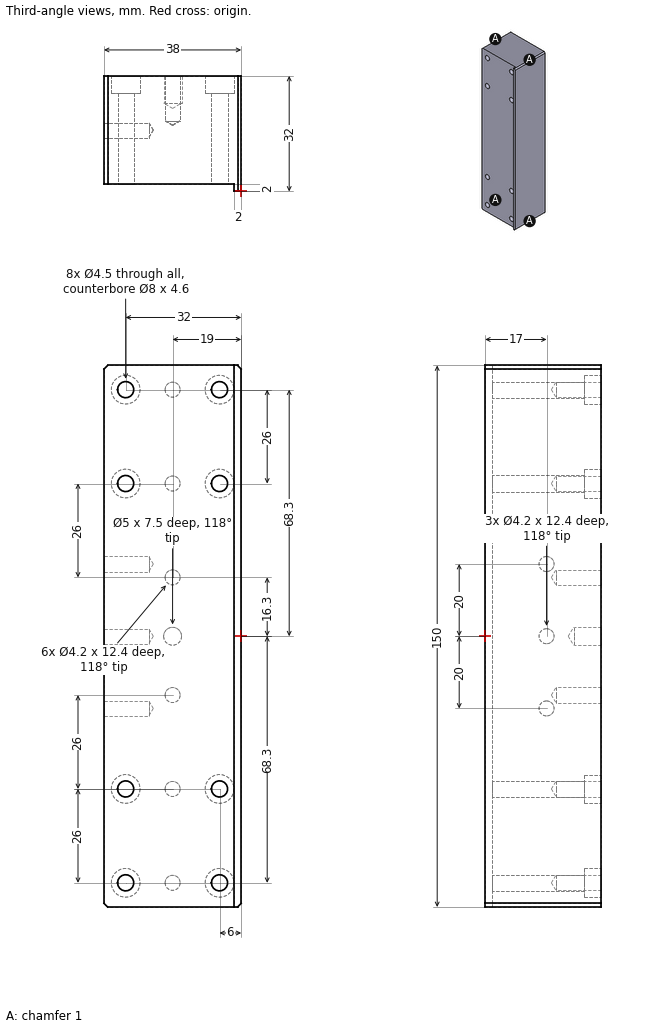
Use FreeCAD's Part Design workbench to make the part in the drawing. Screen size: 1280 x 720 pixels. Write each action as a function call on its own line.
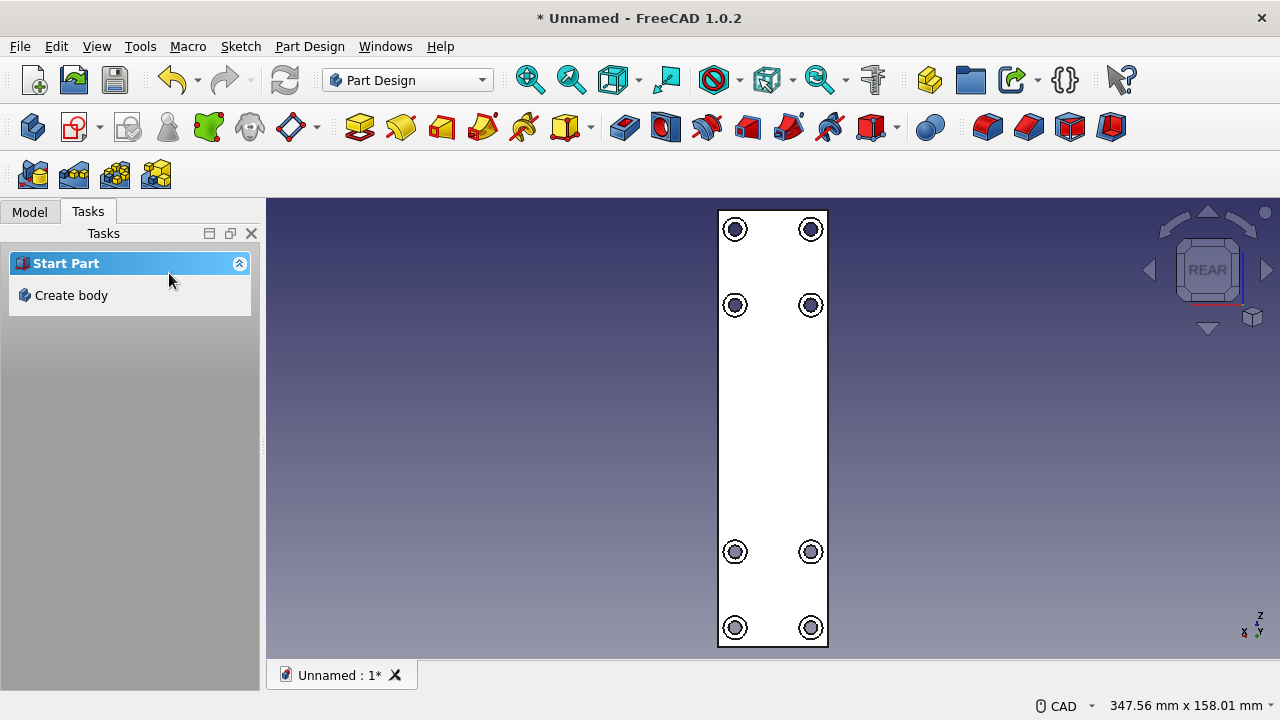
click(773, 365)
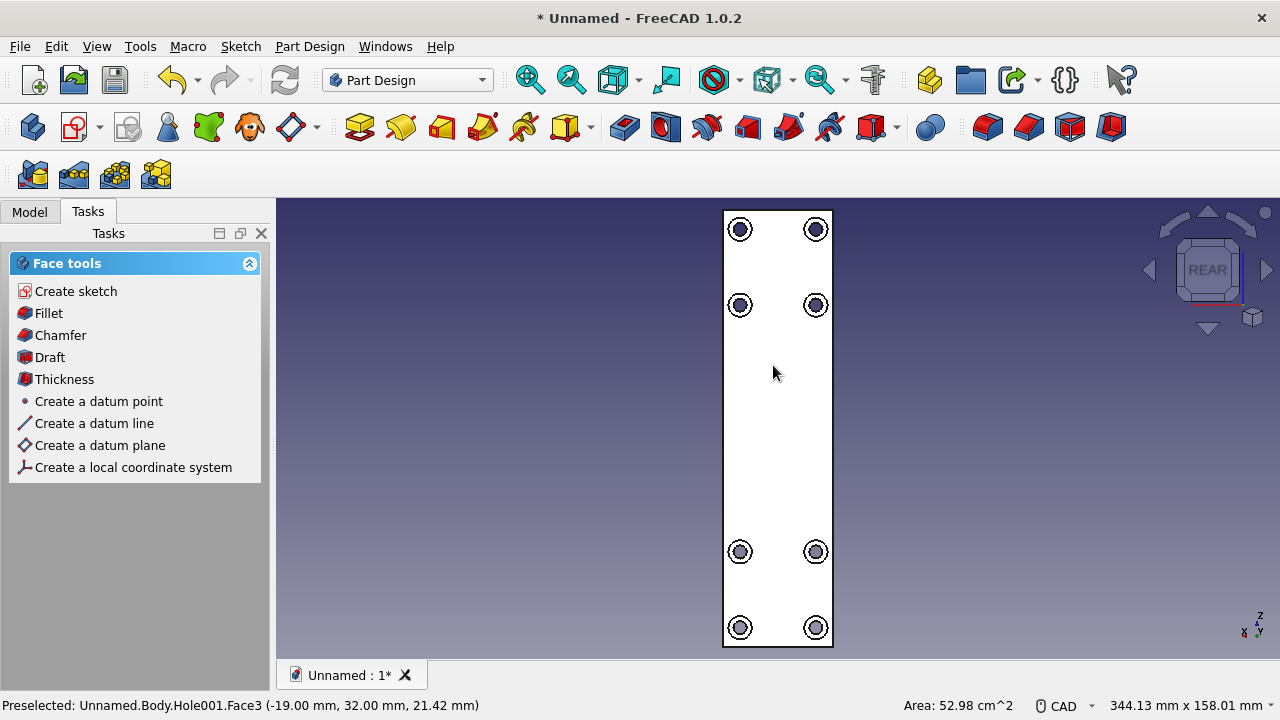
click(74, 128)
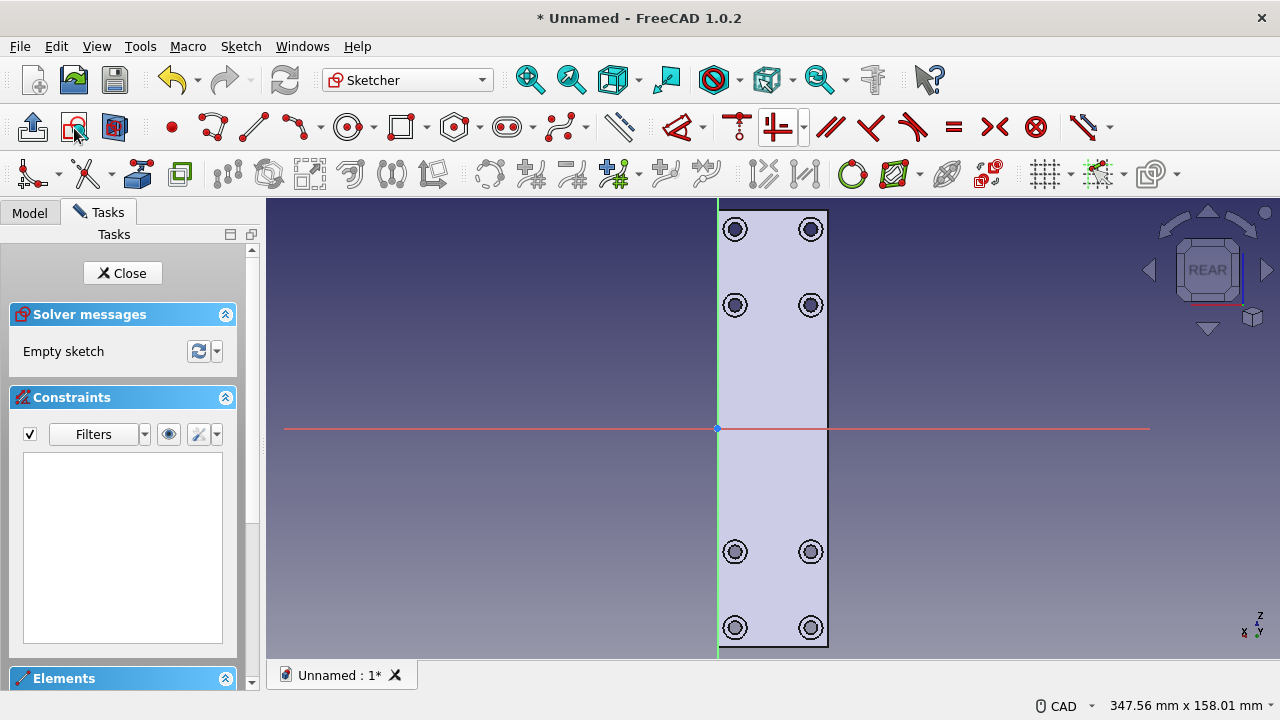
scroll(615, 428, down, 2)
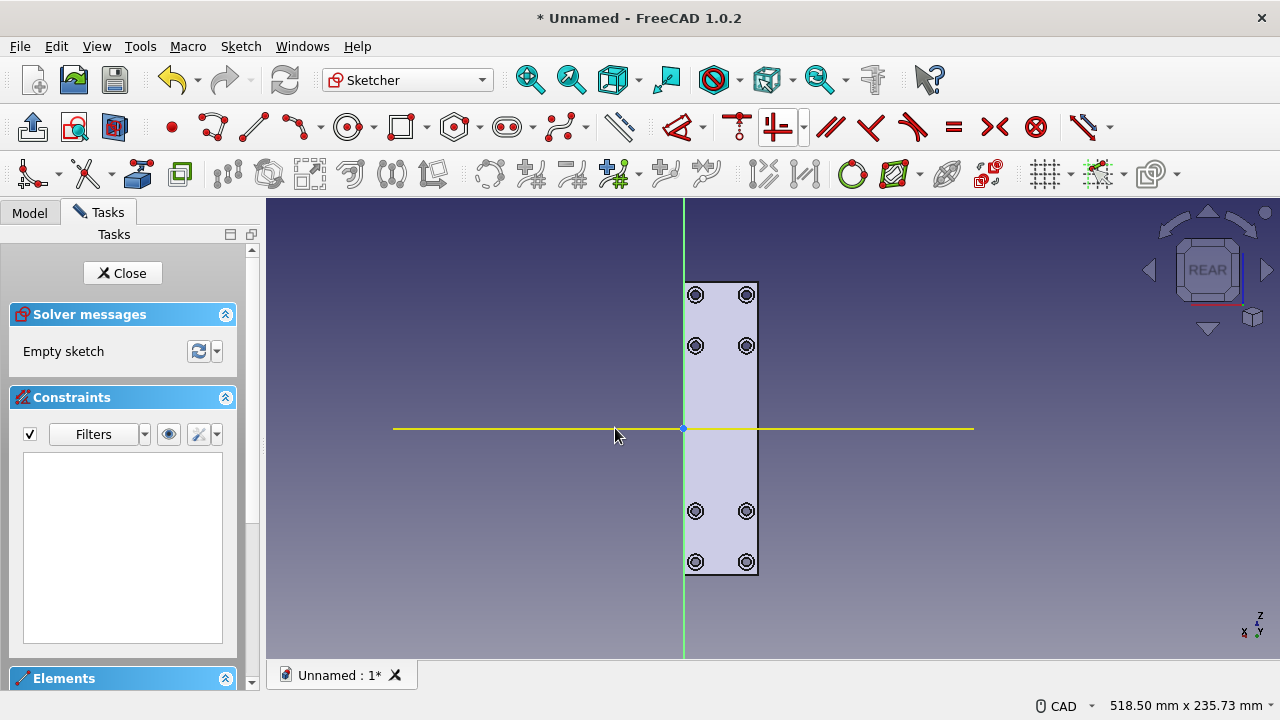
click(348, 128)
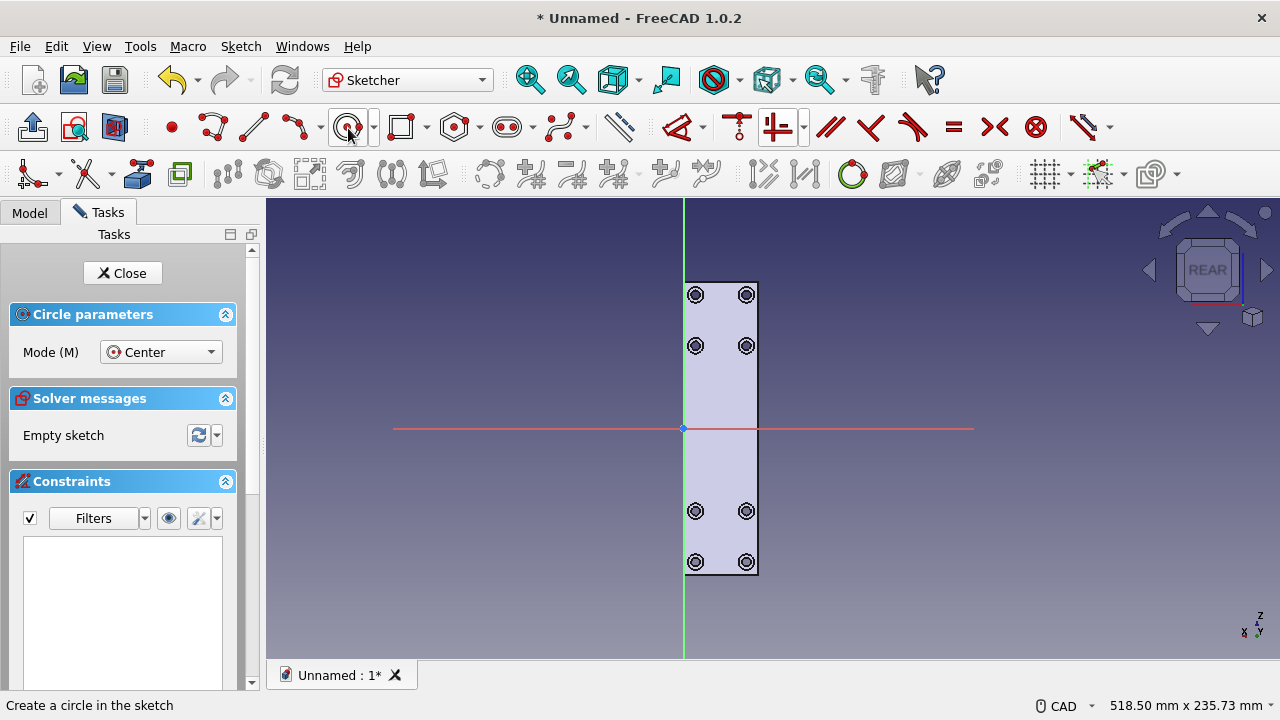
scroll(721, 397, up, 9)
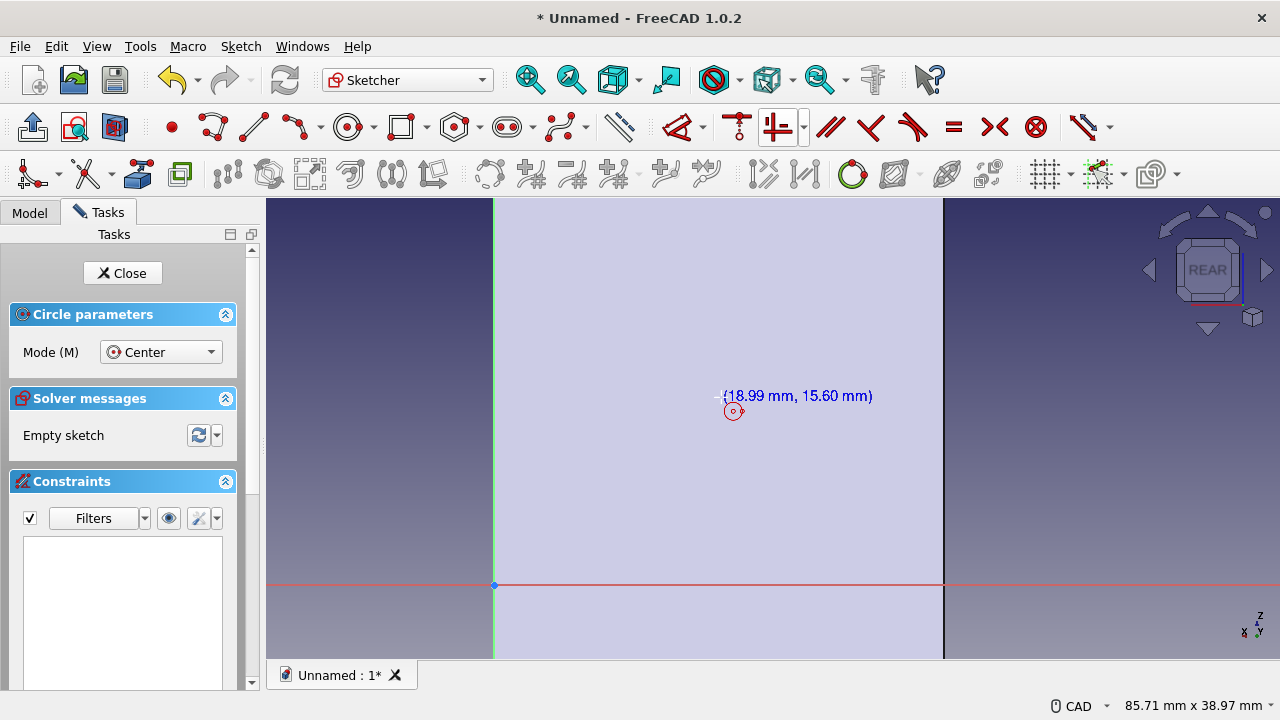
scroll(721, 397, down, 9)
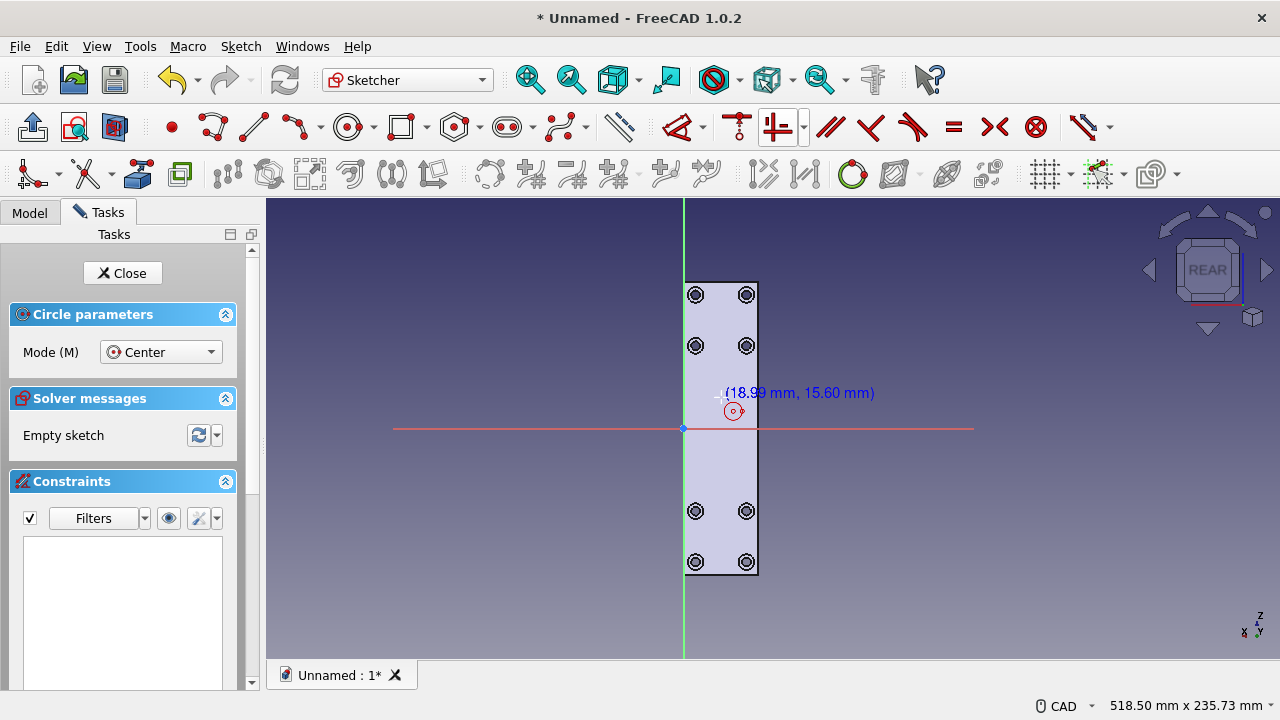
click(721, 397)
move(724, 394)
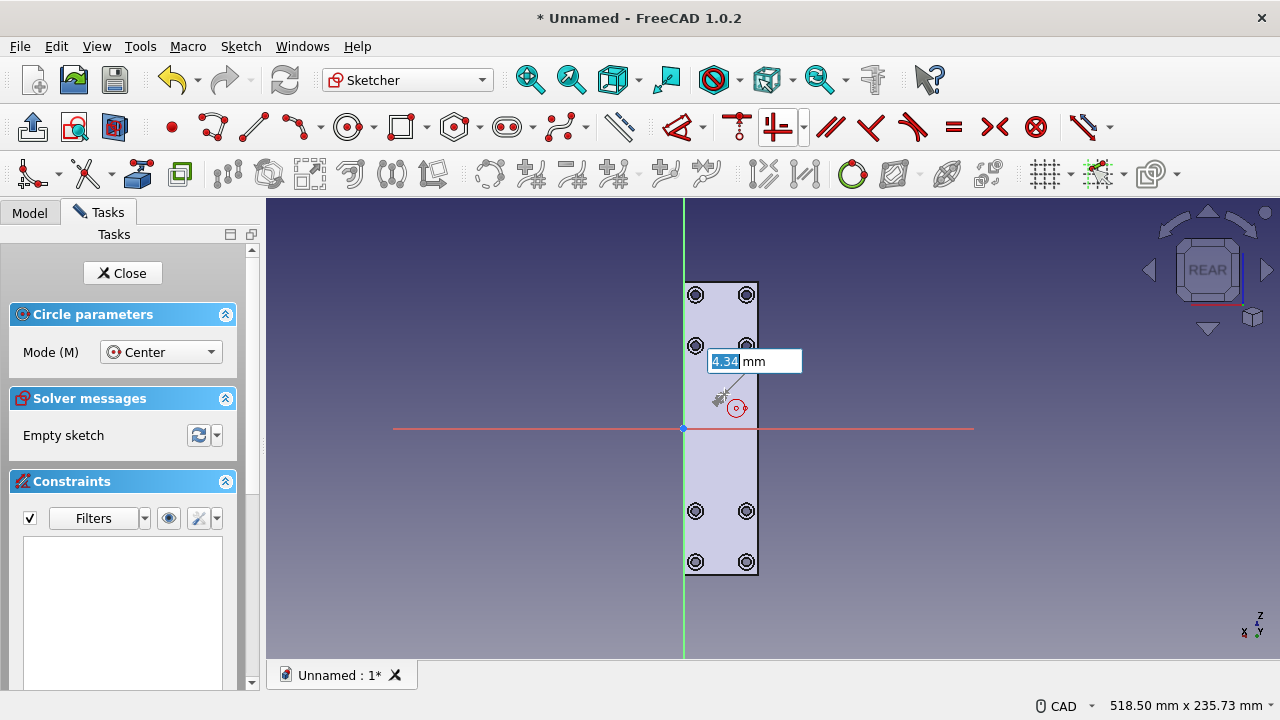
text(4.2)
key(Return)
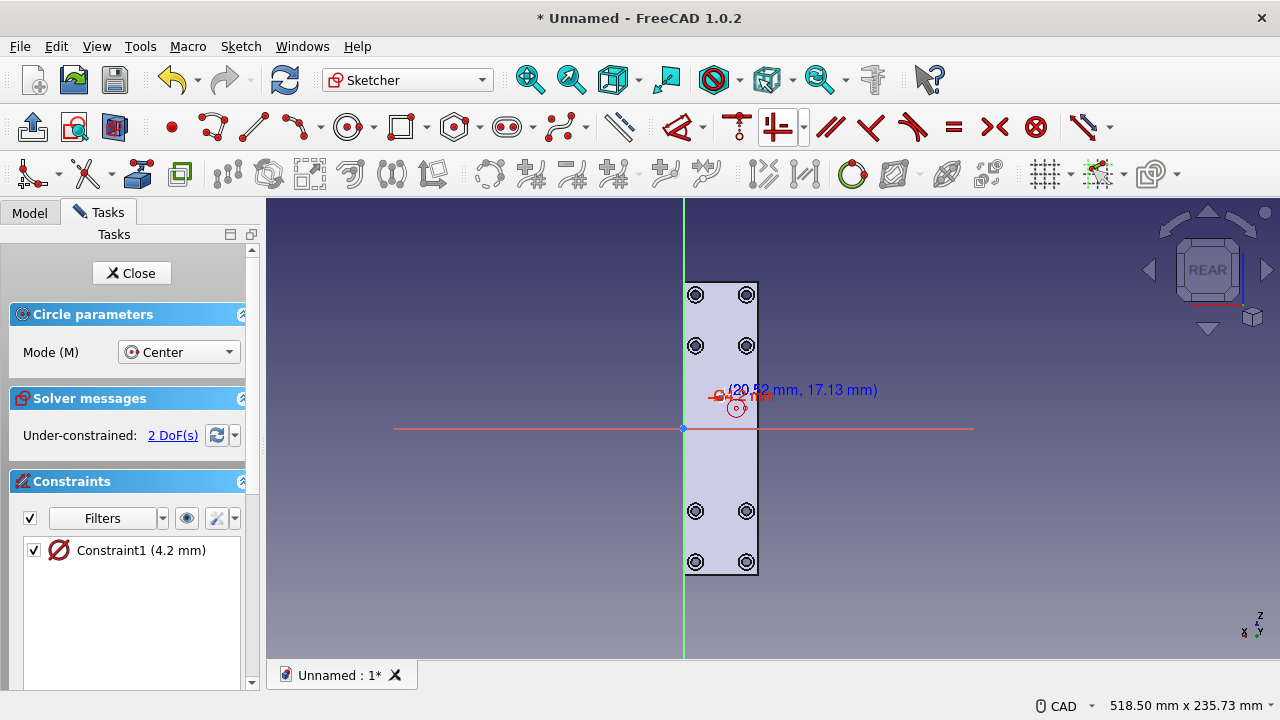
scroll(721, 562, up, 9)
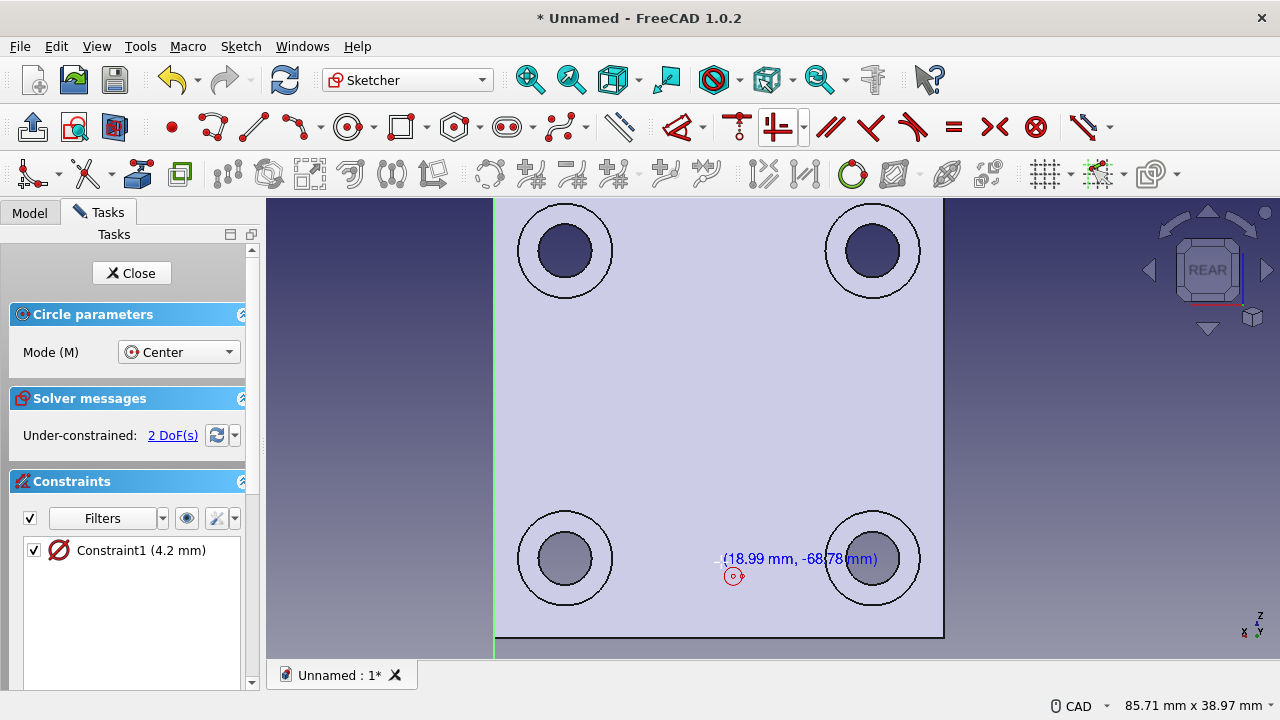
scroll(721, 563, down, 9)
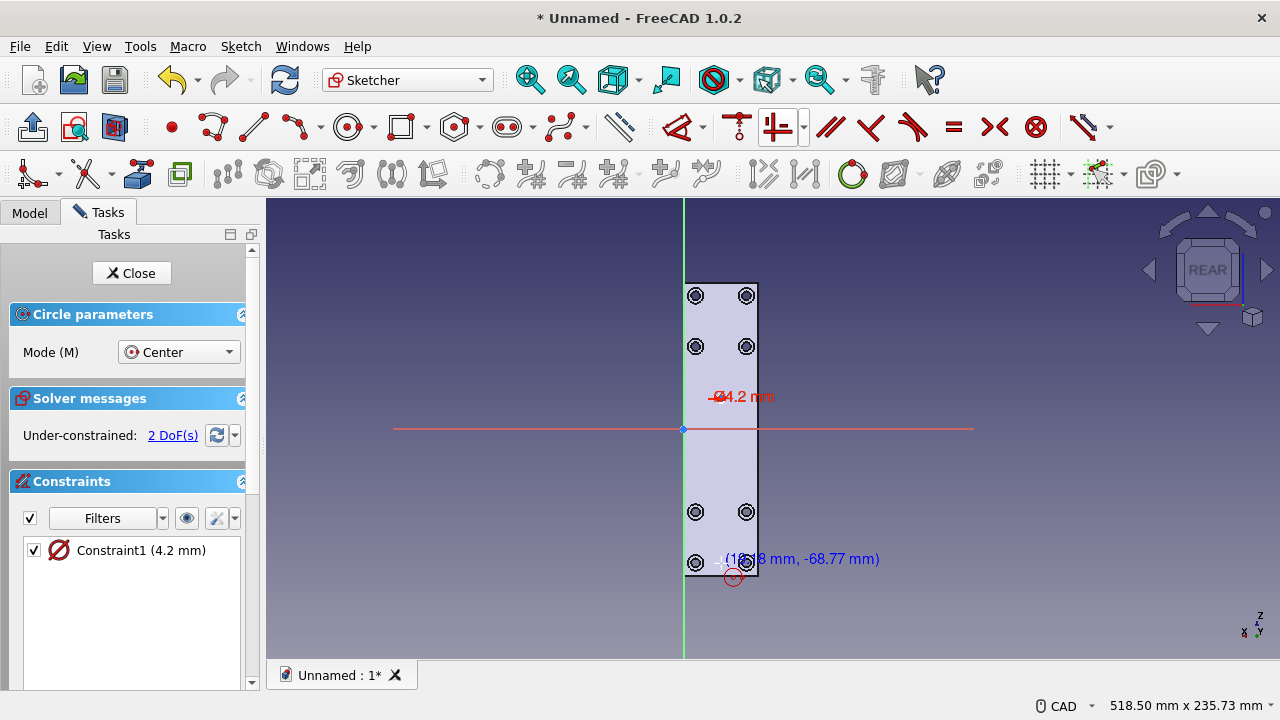
click(721, 563)
move(724, 560)